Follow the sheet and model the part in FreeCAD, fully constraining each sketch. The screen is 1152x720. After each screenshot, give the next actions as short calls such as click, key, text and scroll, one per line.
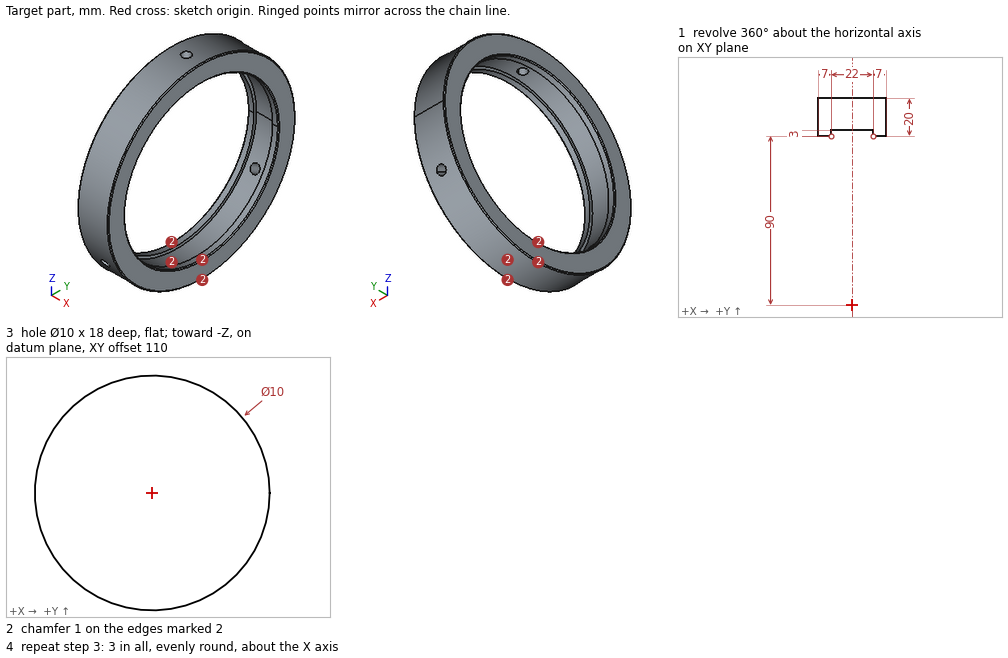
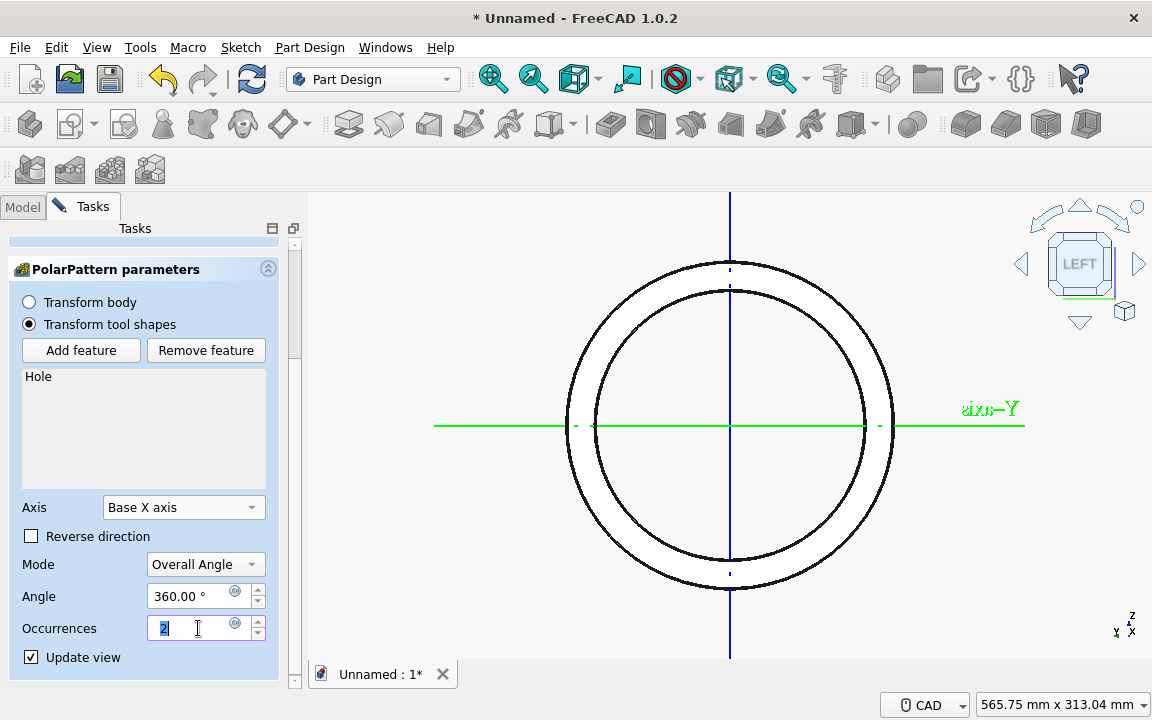
text(3)
key(Tab)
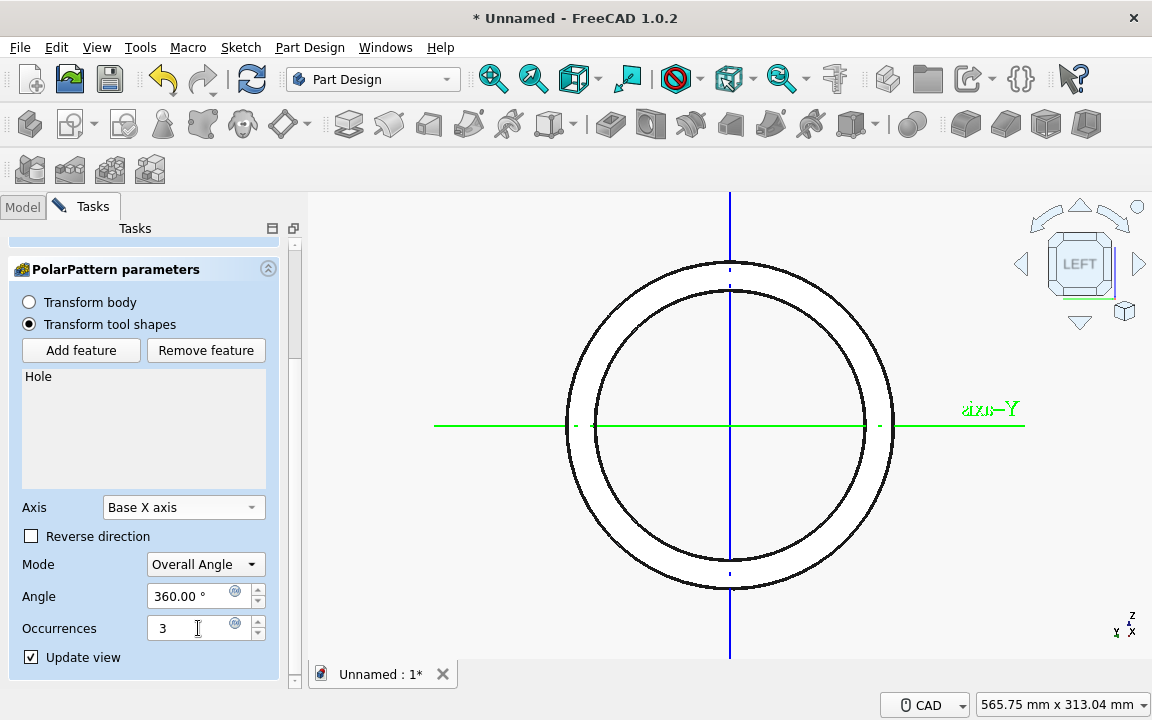
scroll(295, 463, up, 4)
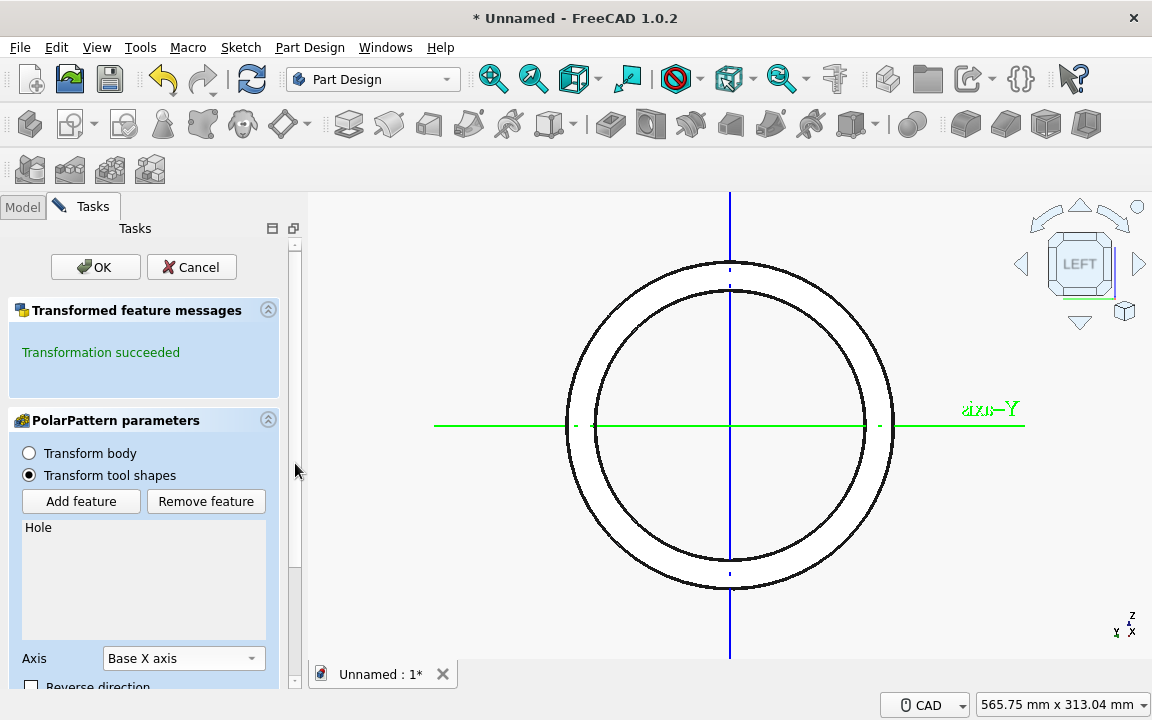
click(96, 267)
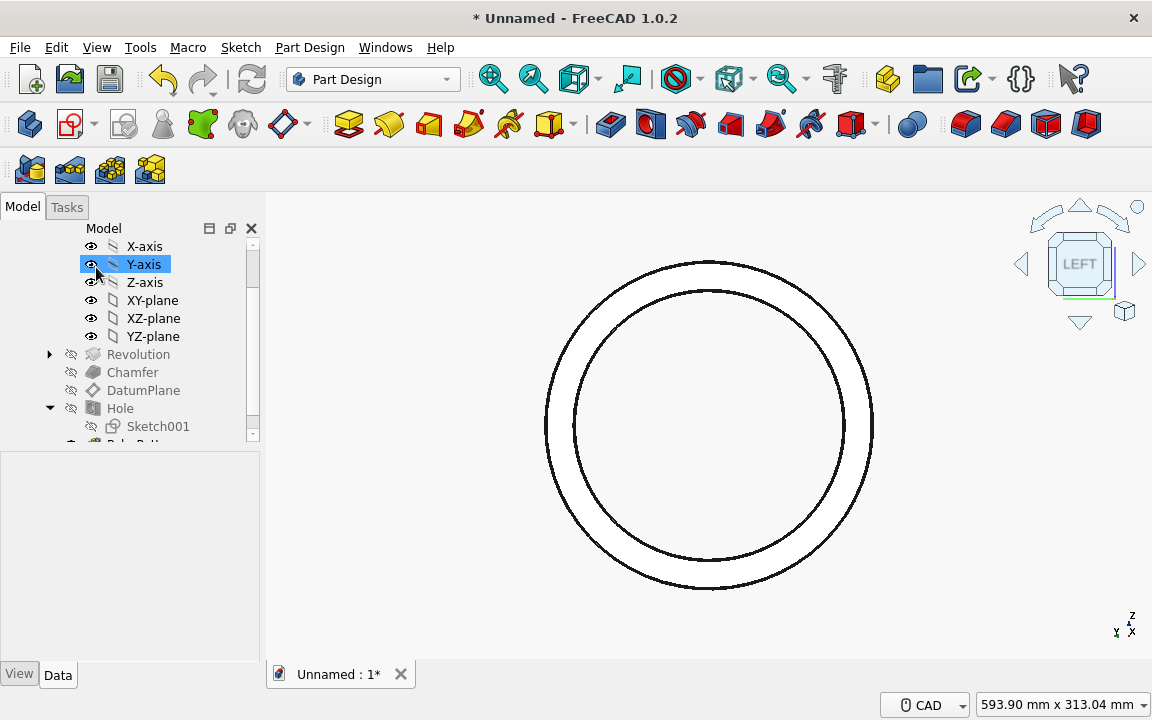
key(0)